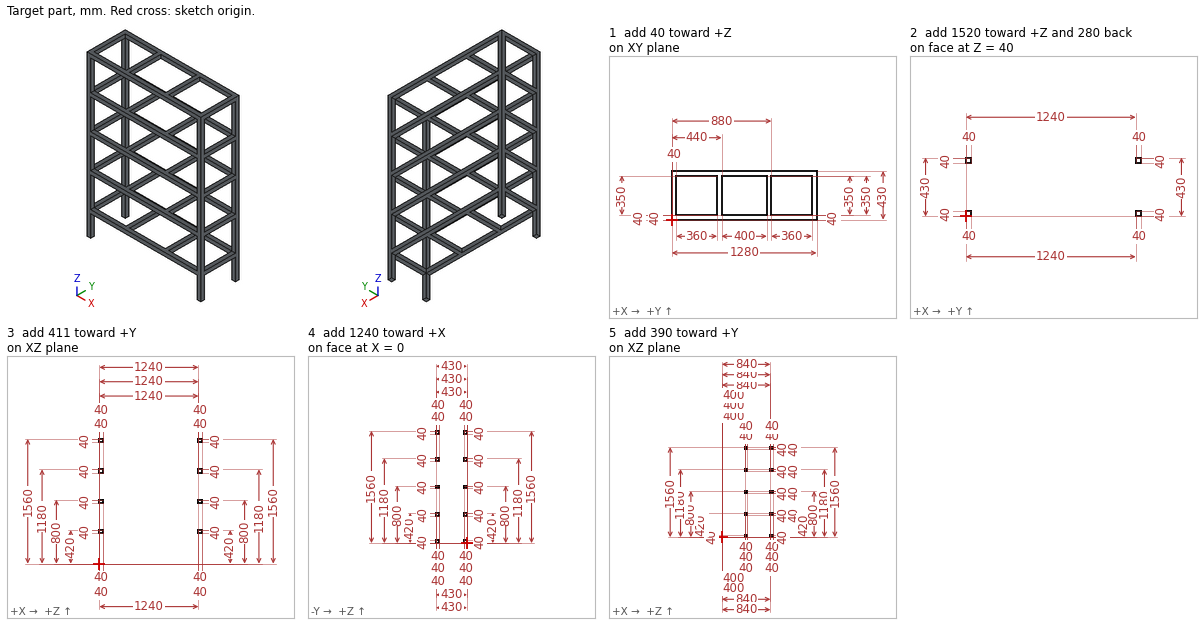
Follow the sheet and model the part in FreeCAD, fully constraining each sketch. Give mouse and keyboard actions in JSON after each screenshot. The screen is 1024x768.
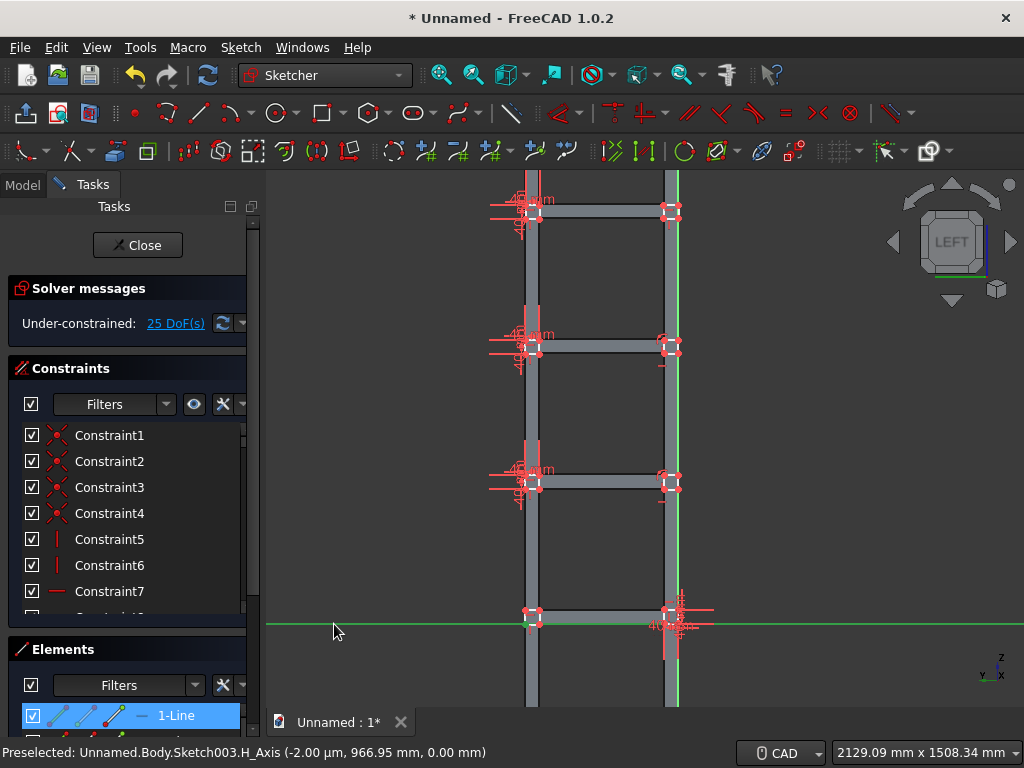
{"action": "left_click", "coordinate": [614, 114]}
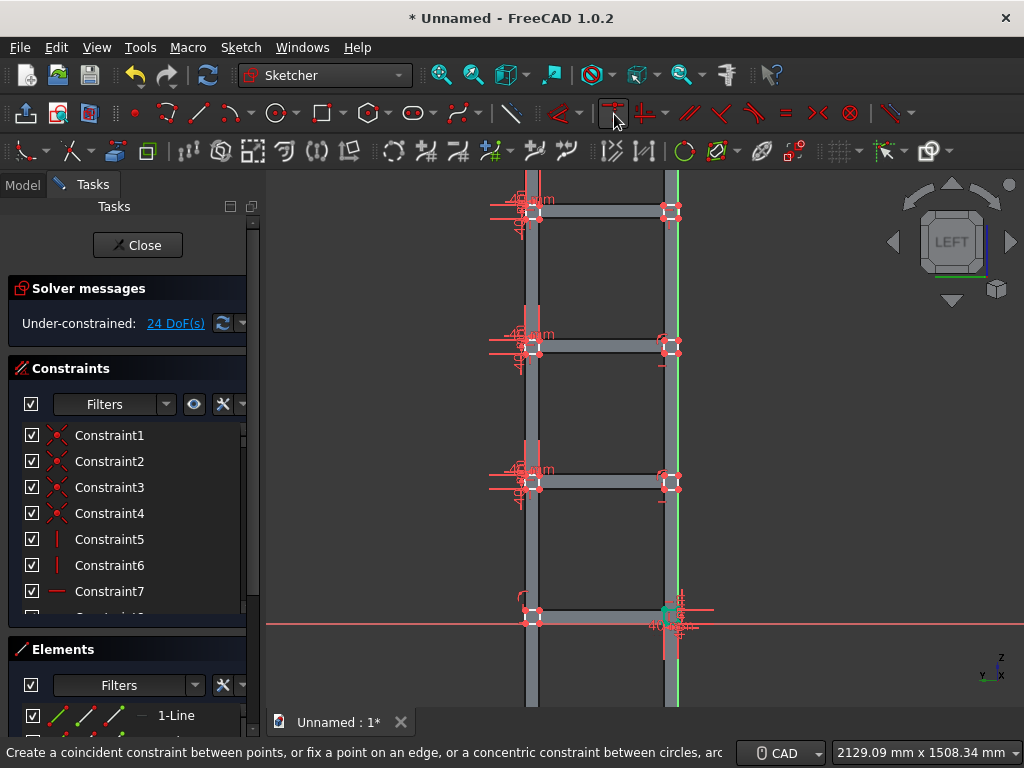
{"action": "left_click", "coordinate": [679, 219]}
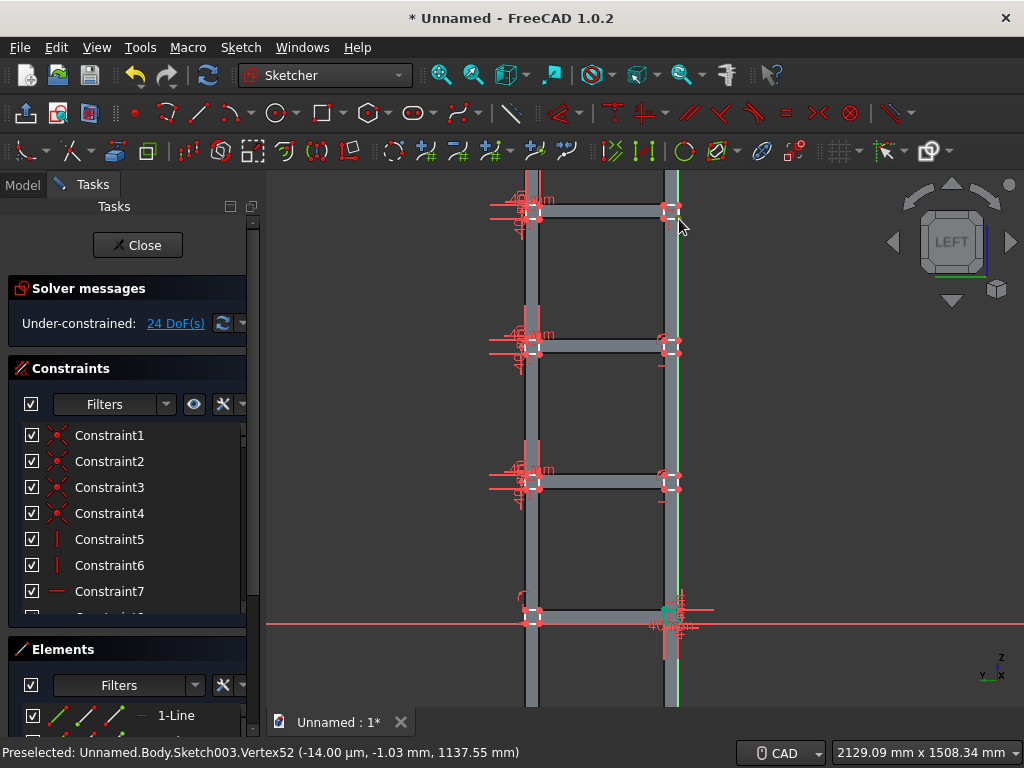
{"action": "left_click", "coordinate": [678, 576]}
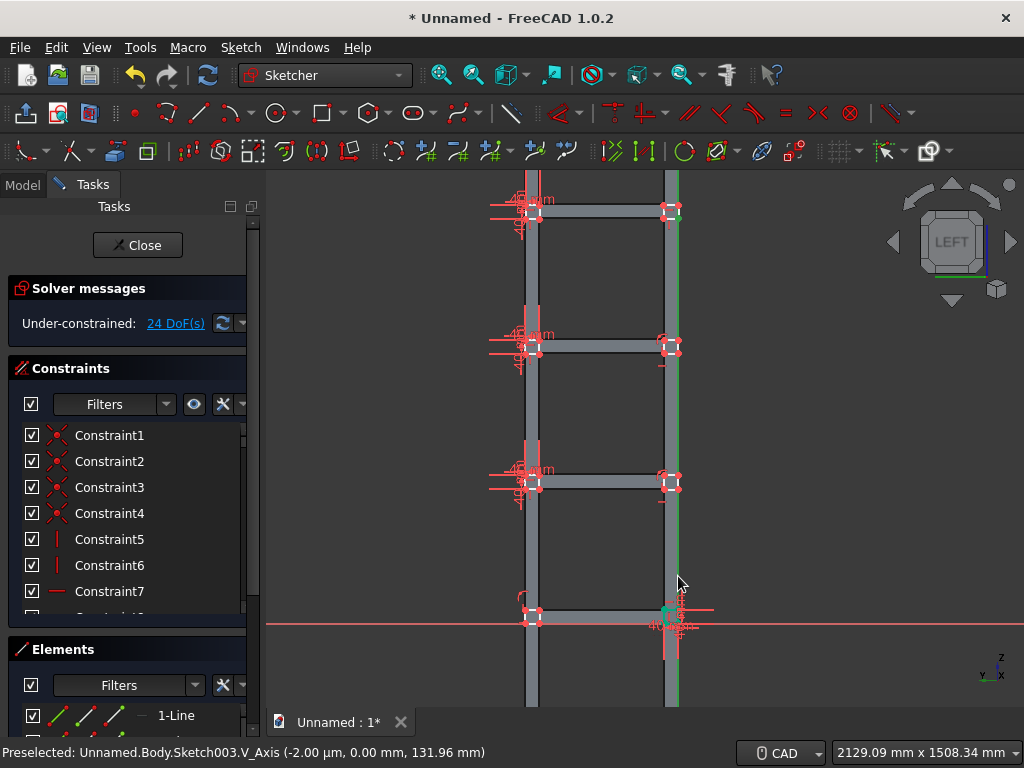
{"action": "left_click", "coordinate": [614, 114]}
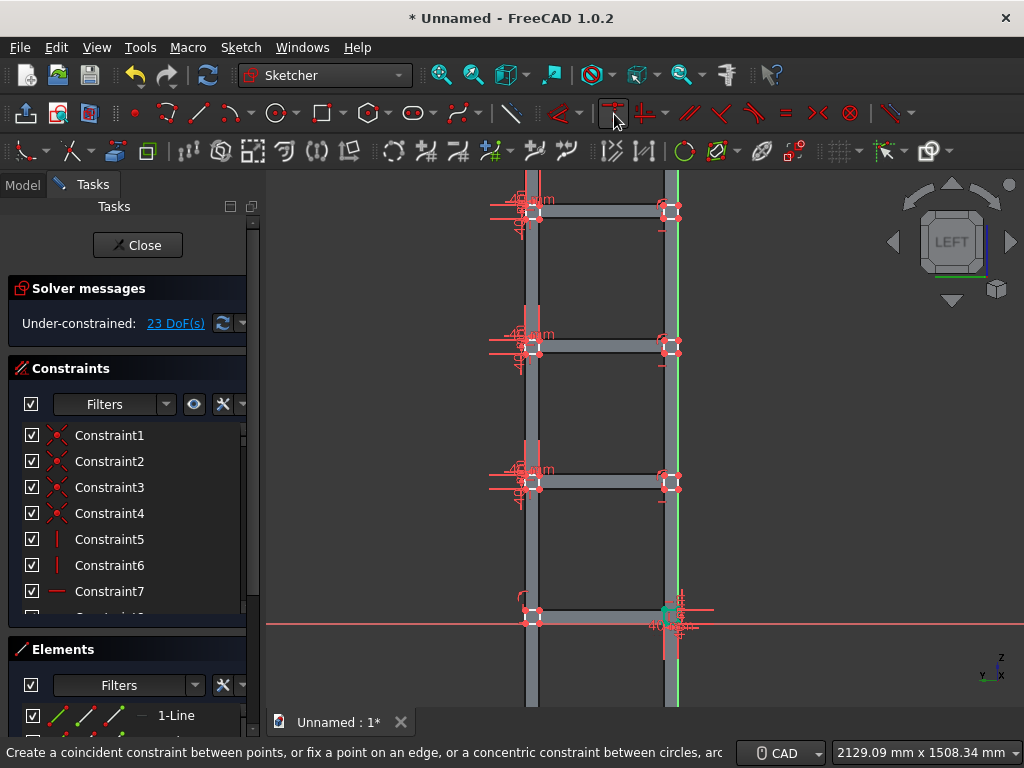
{"action": "left_click", "coordinate": [558, 114]}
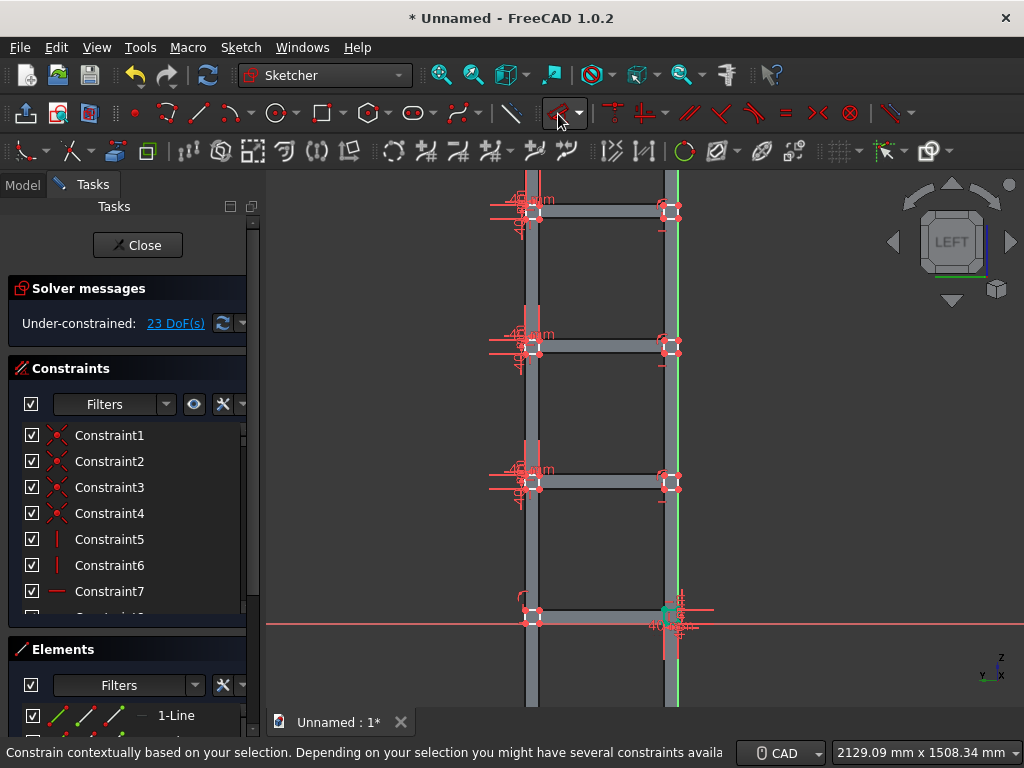
{"action": "scroll", "coordinate": [525, 617], "scroll_direction": "up", "scroll_amount": 6}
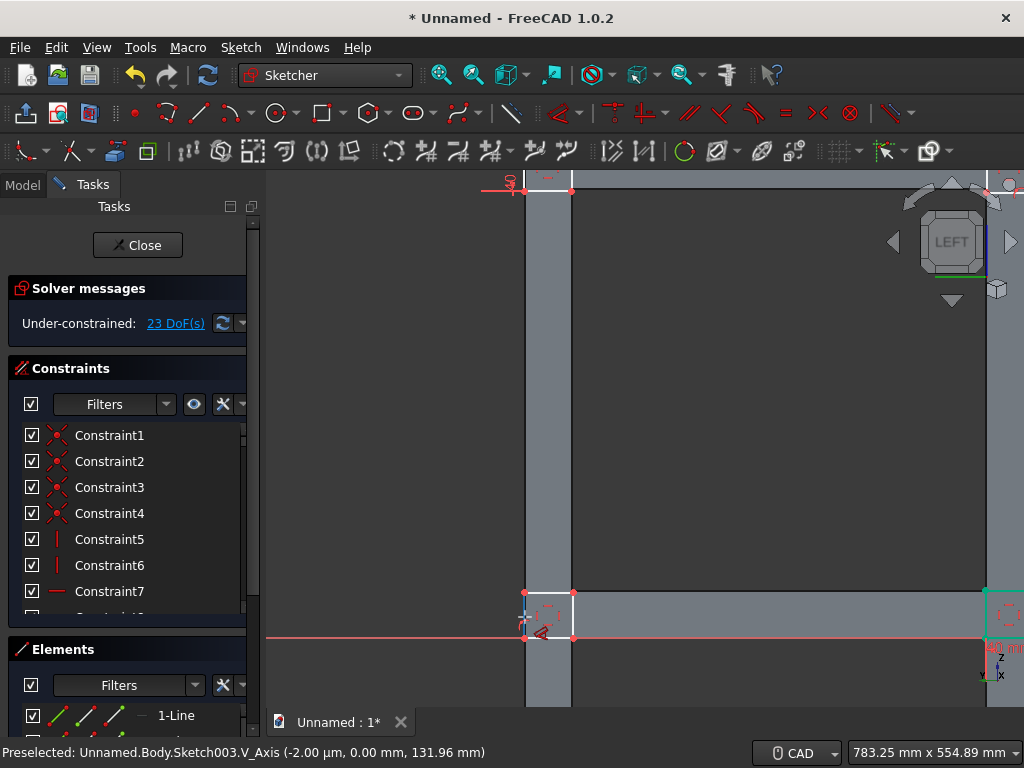
{"action": "left_click", "coordinate": [524, 615]}
{"action": "left_click", "coordinate": [490, 615]}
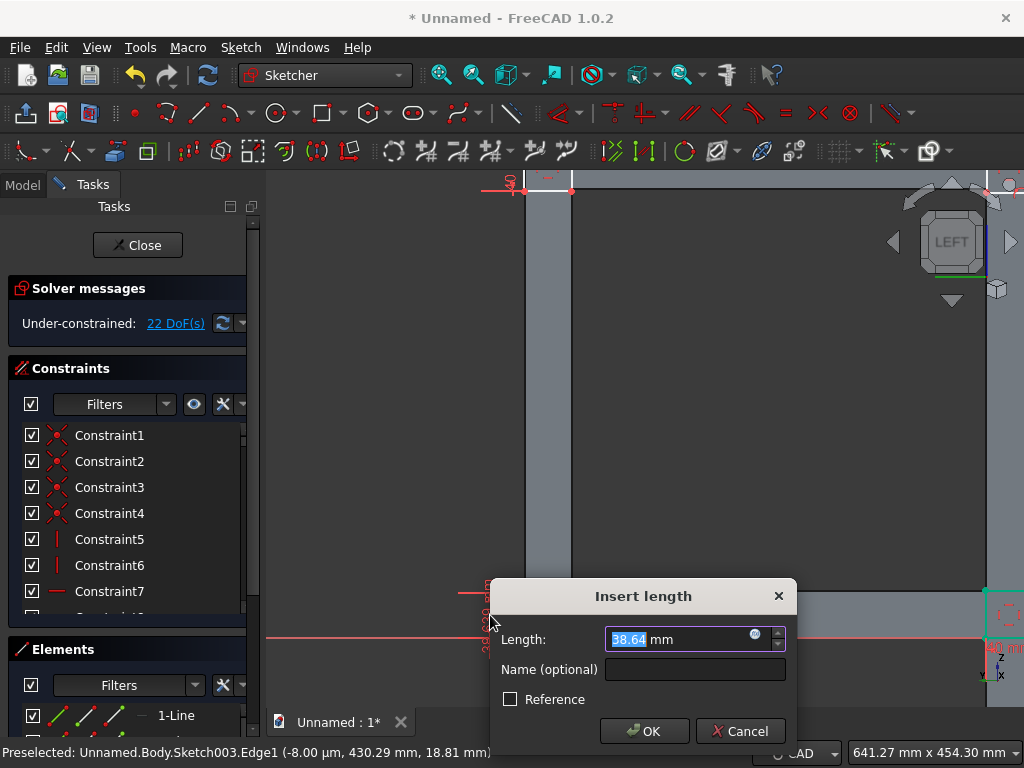
{"action": "type", "text": "40"}
{"action": "key", "text": "Return"}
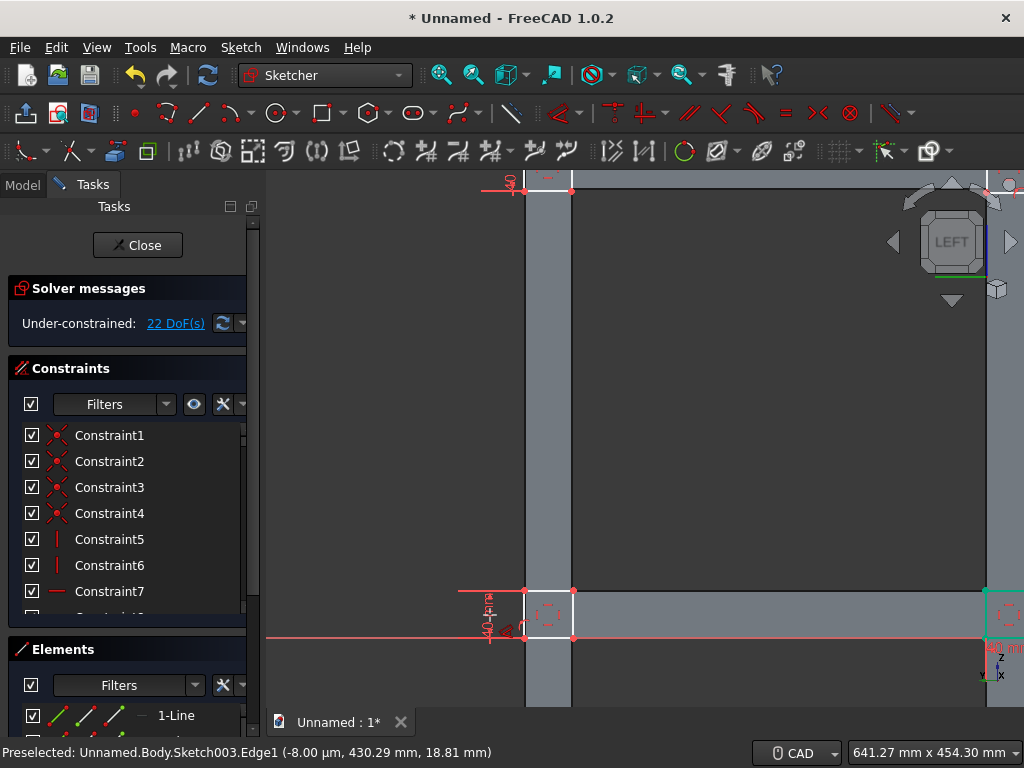
{"action": "left_click", "coordinate": [539, 638]}
{"action": "left_click", "coordinate": [549, 672]}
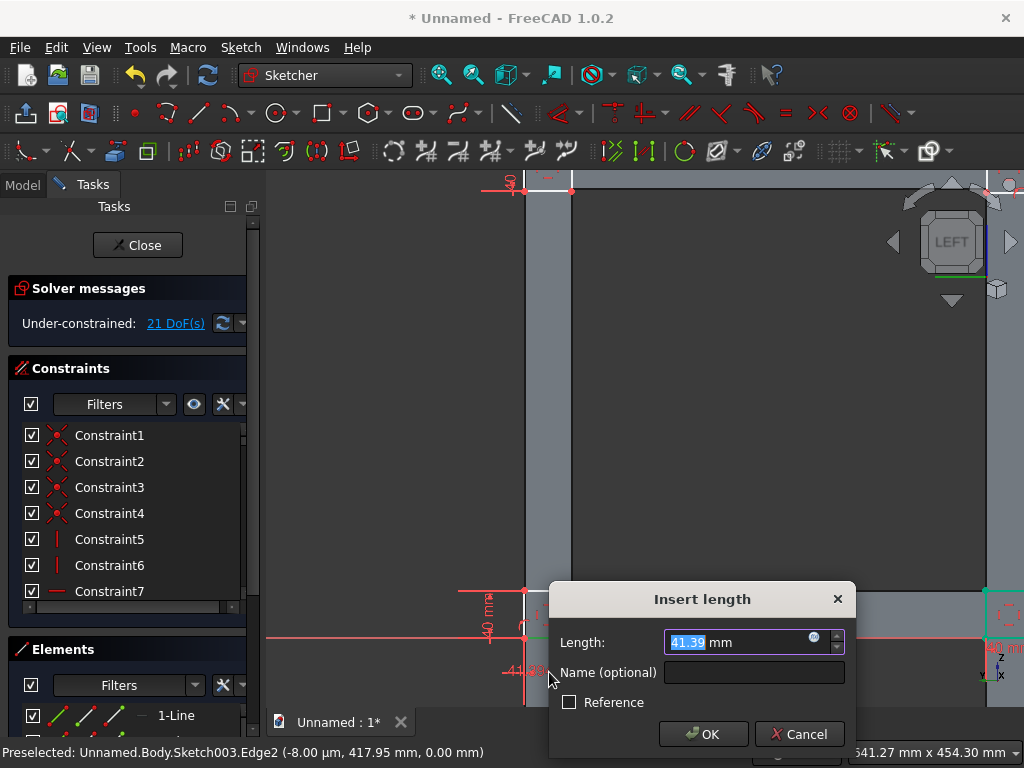
{"action": "type", "text": "40"}
{"action": "key", "text": "Return"}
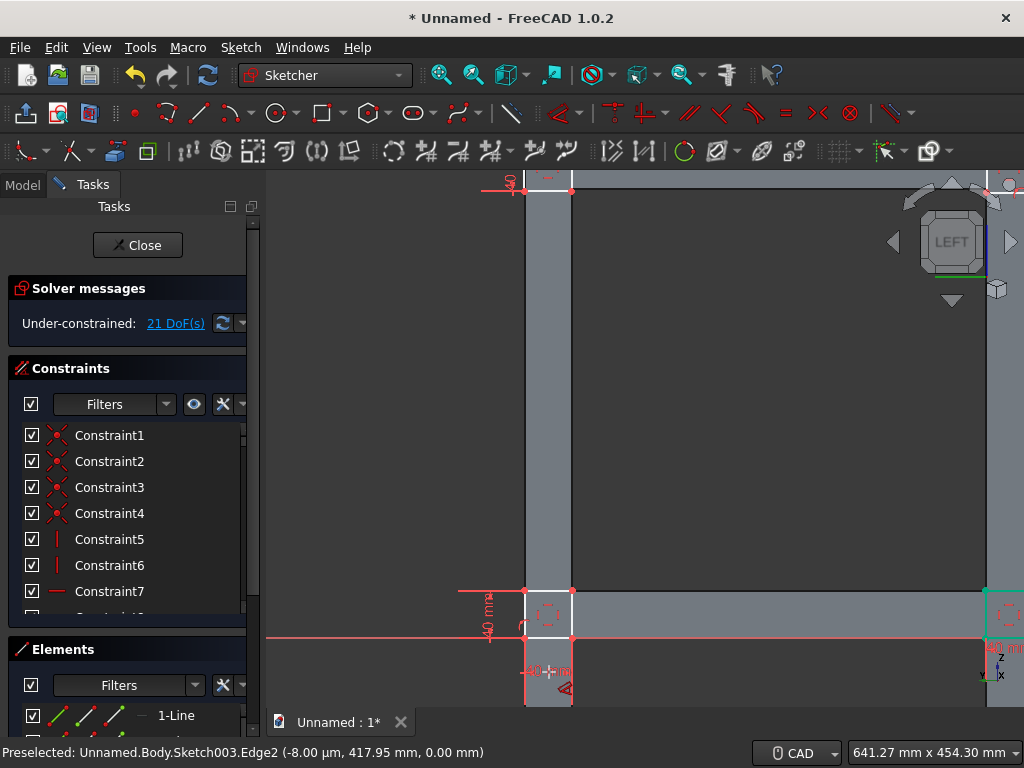
{"action": "scroll", "coordinate": [525, 621], "scroll_direction": "down", "scroll_amount": 8}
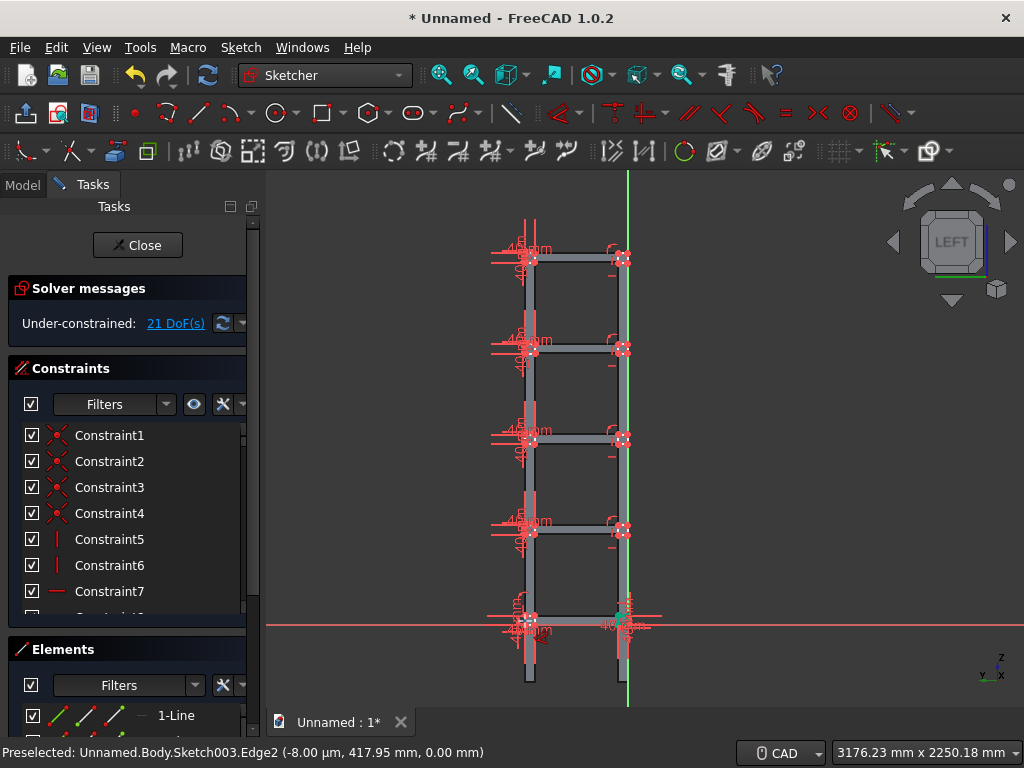
{"action": "scroll", "coordinate": [618, 528], "scroll_direction": "up", "scroll_amount": 8}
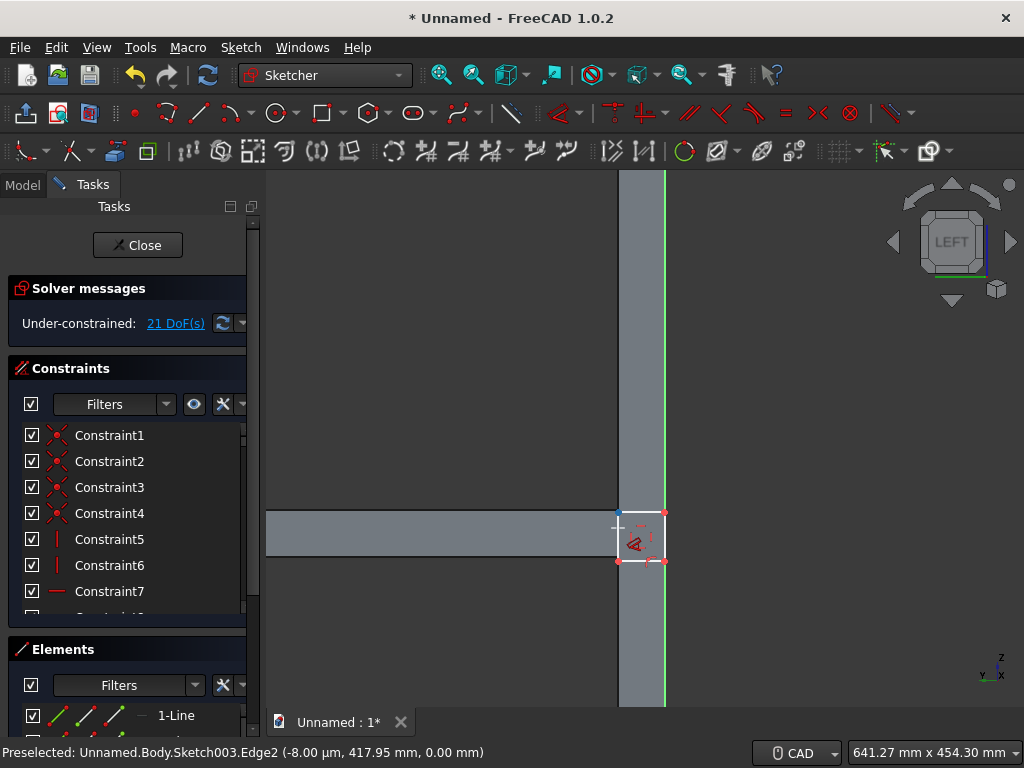
{"action": "left_click", "coordinate": [618, 527]}
{"action": "left_click", "coordinate": [584, 537]}